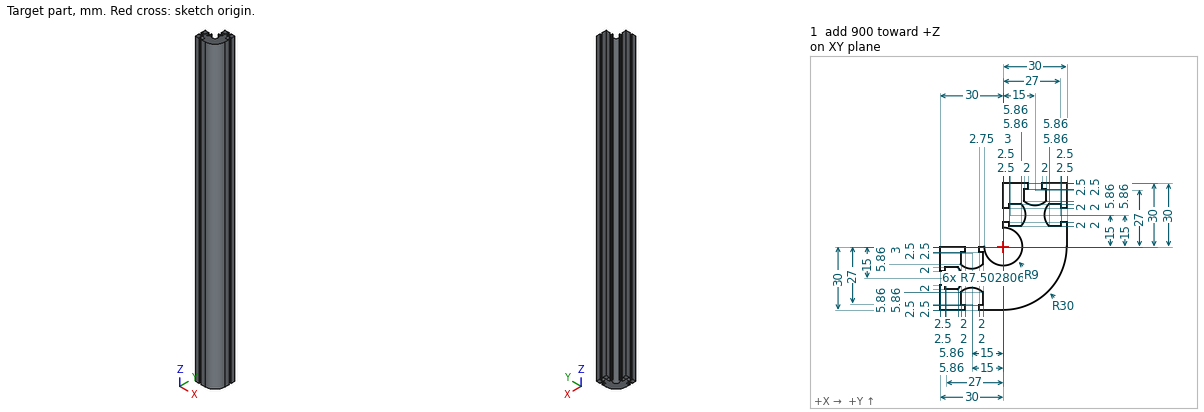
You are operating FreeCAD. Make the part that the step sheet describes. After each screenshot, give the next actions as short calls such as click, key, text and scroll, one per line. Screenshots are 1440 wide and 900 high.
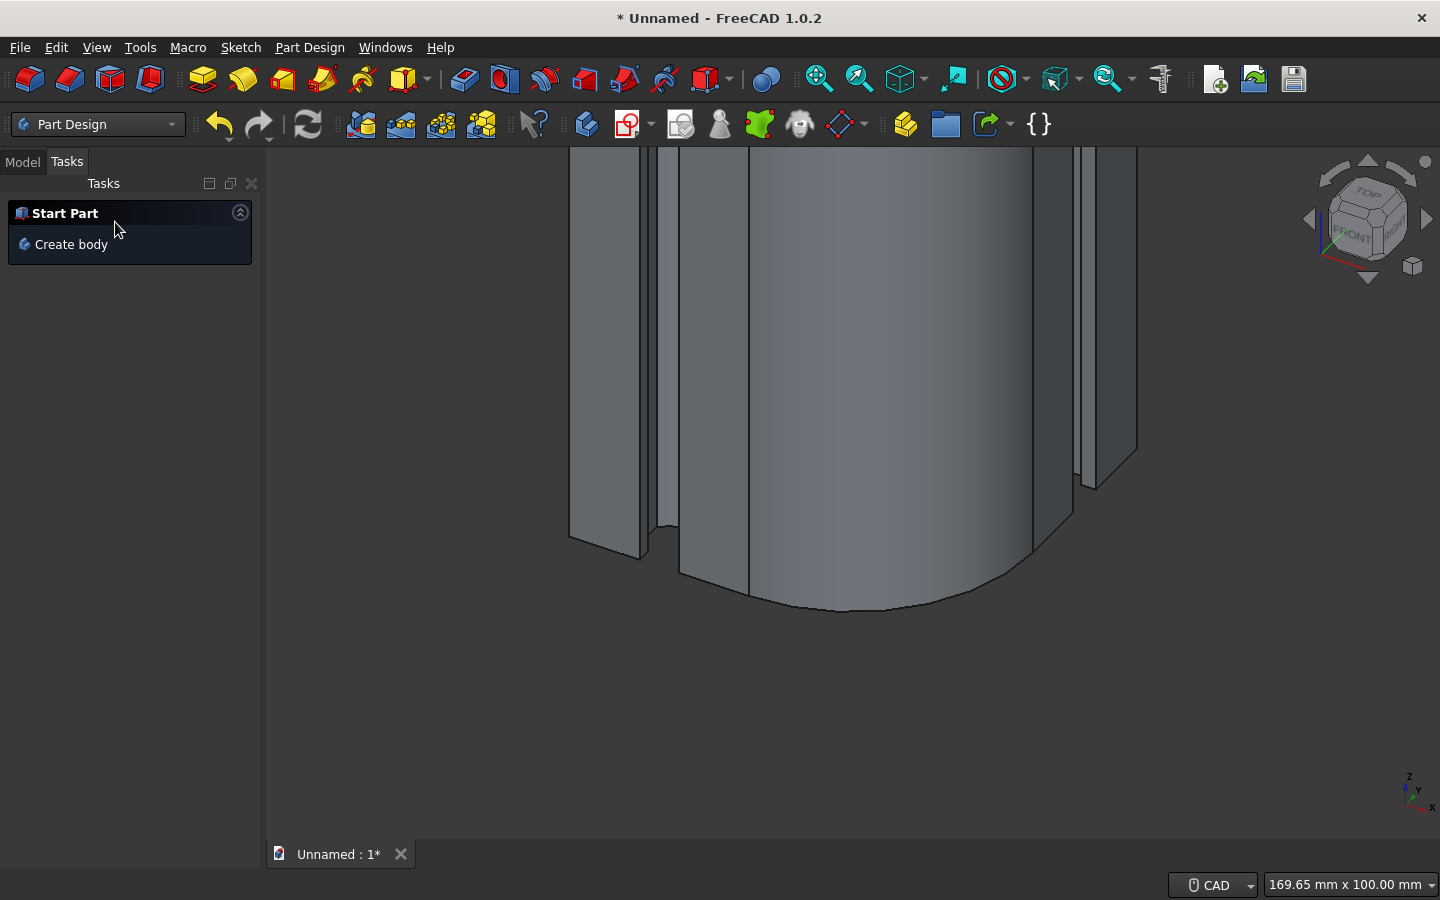
key(0)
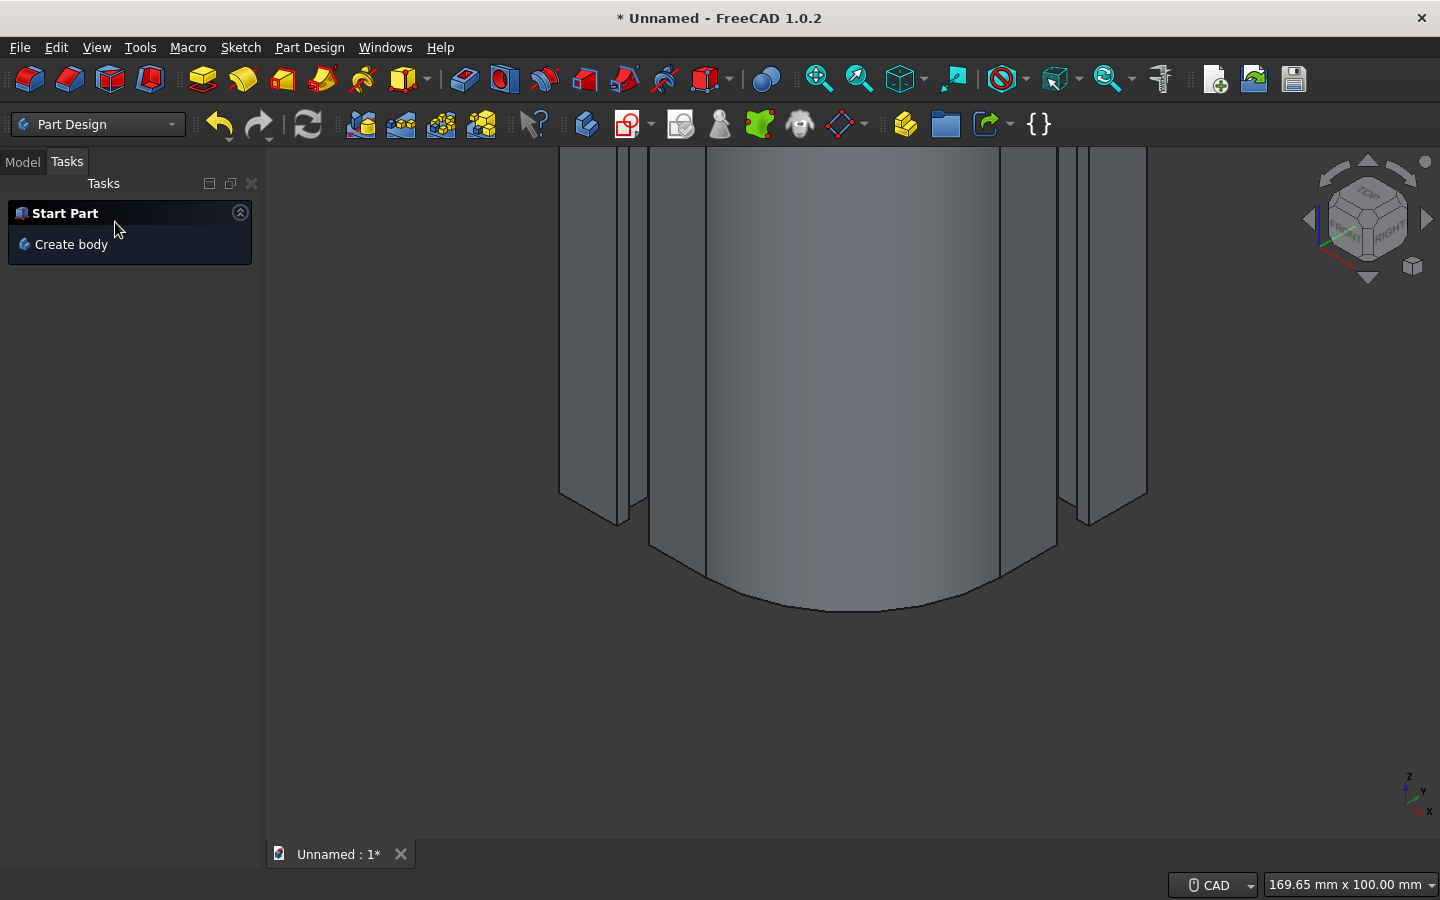
click(820, 80)